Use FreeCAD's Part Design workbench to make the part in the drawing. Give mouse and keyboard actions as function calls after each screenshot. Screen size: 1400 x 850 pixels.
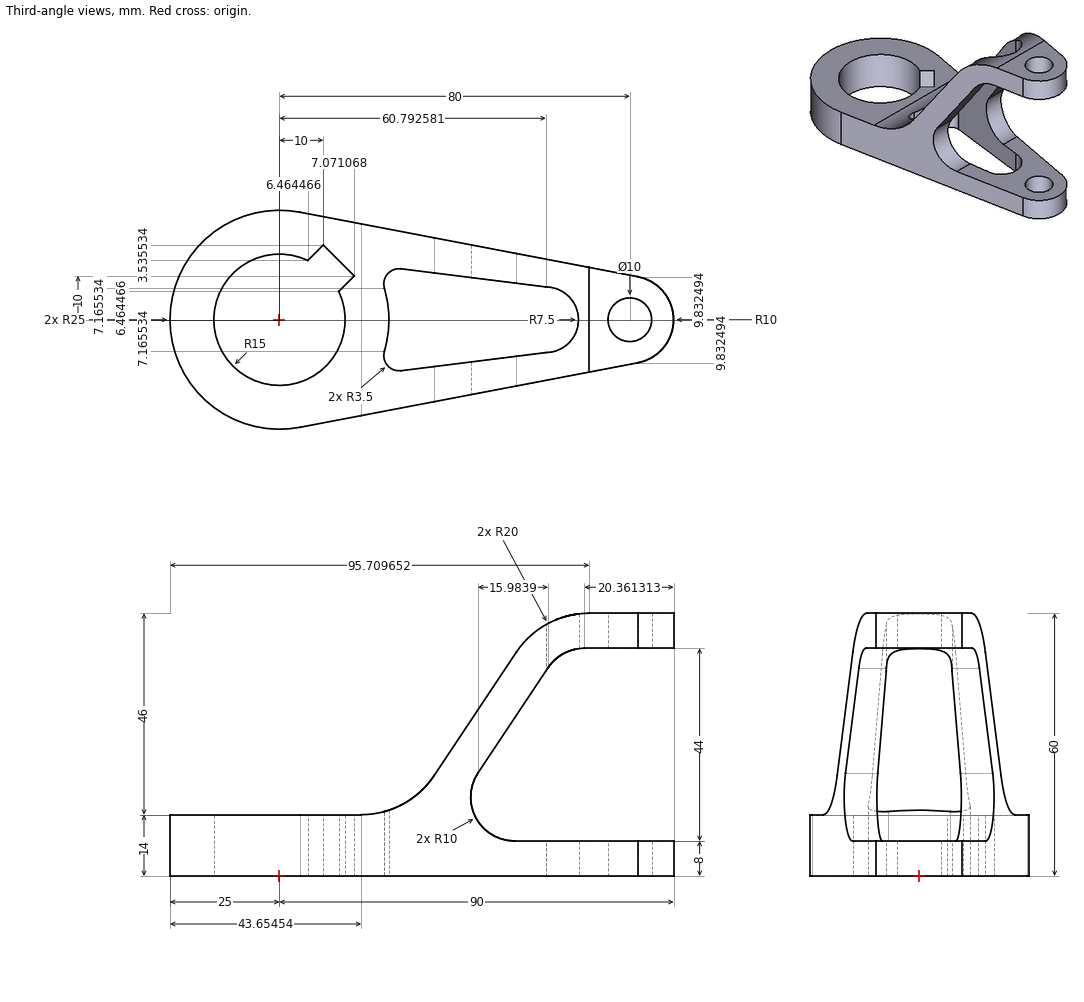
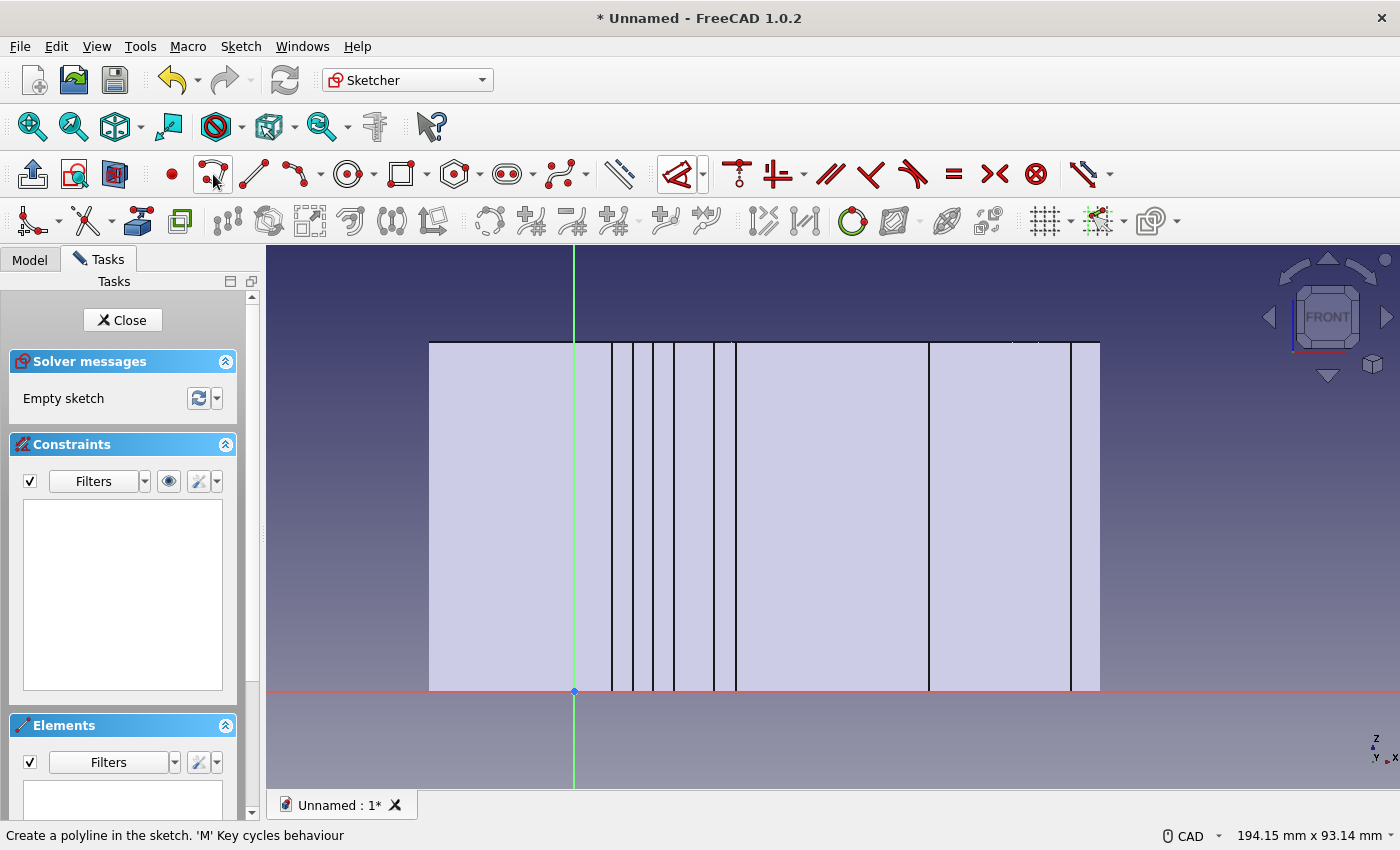
click(683, 610)
click(428, 610)
click(428, 342)
click(987, 342)
right_click(987, 342)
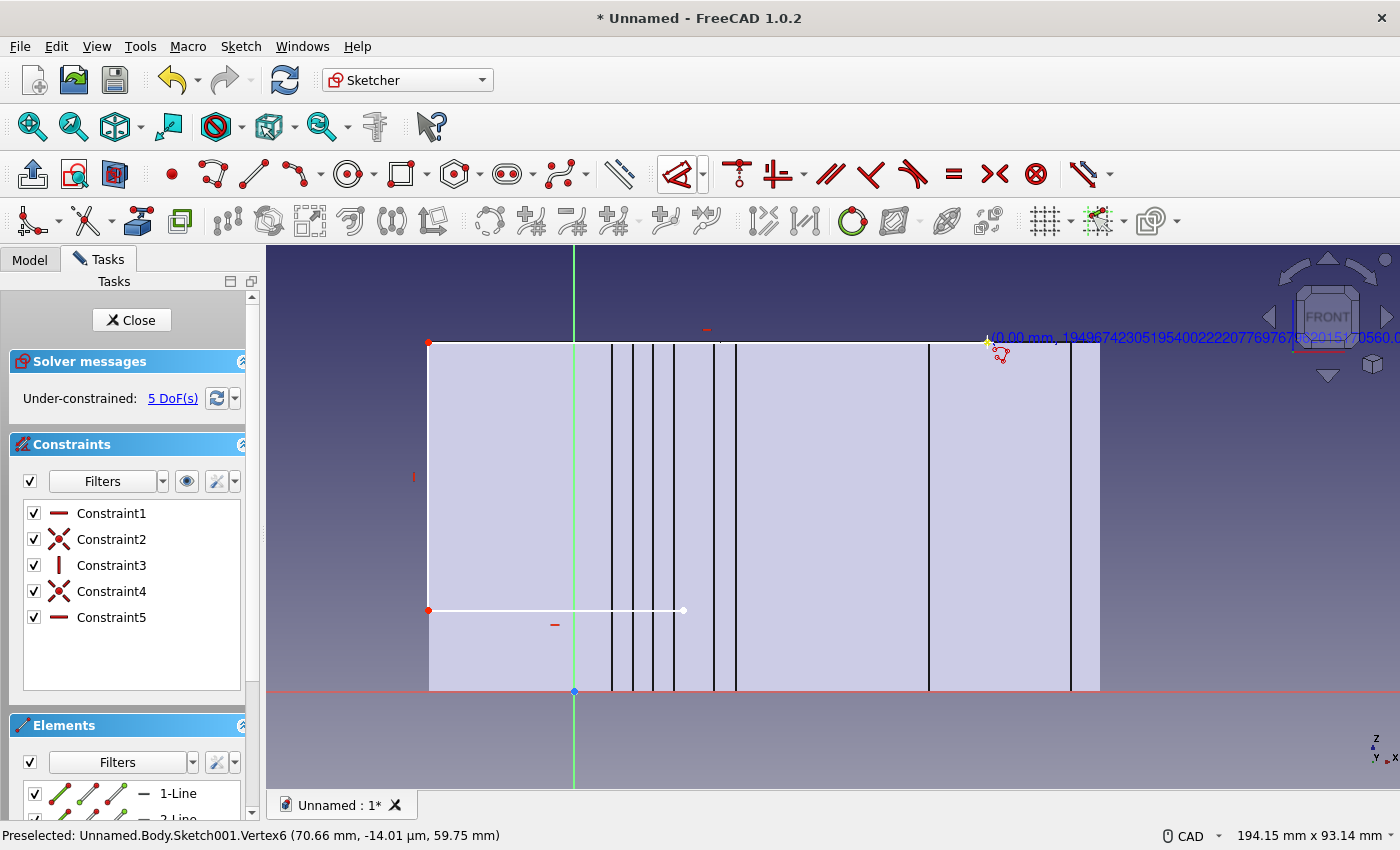
click(254, 174)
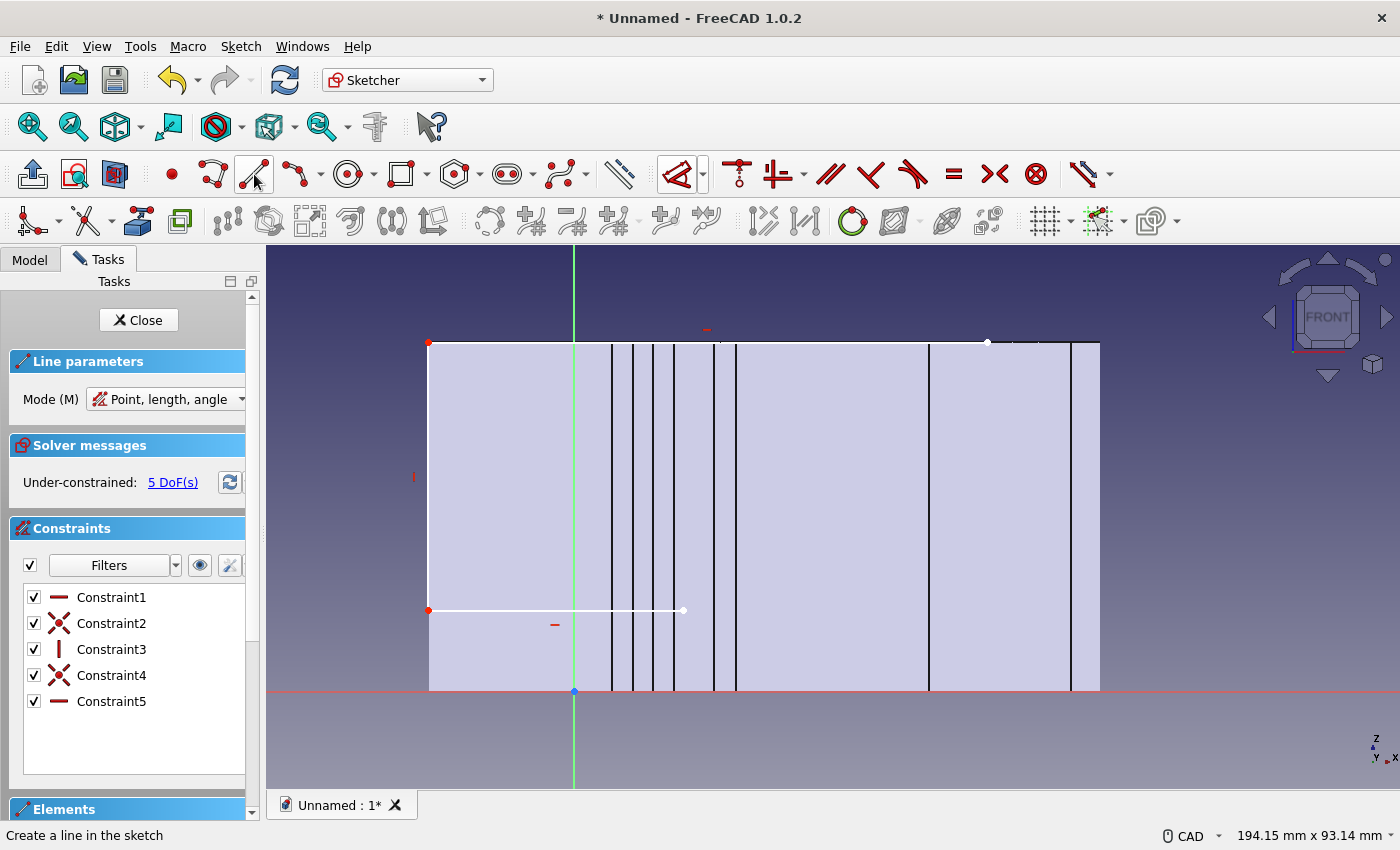
click(890, 394)
click(780, 558)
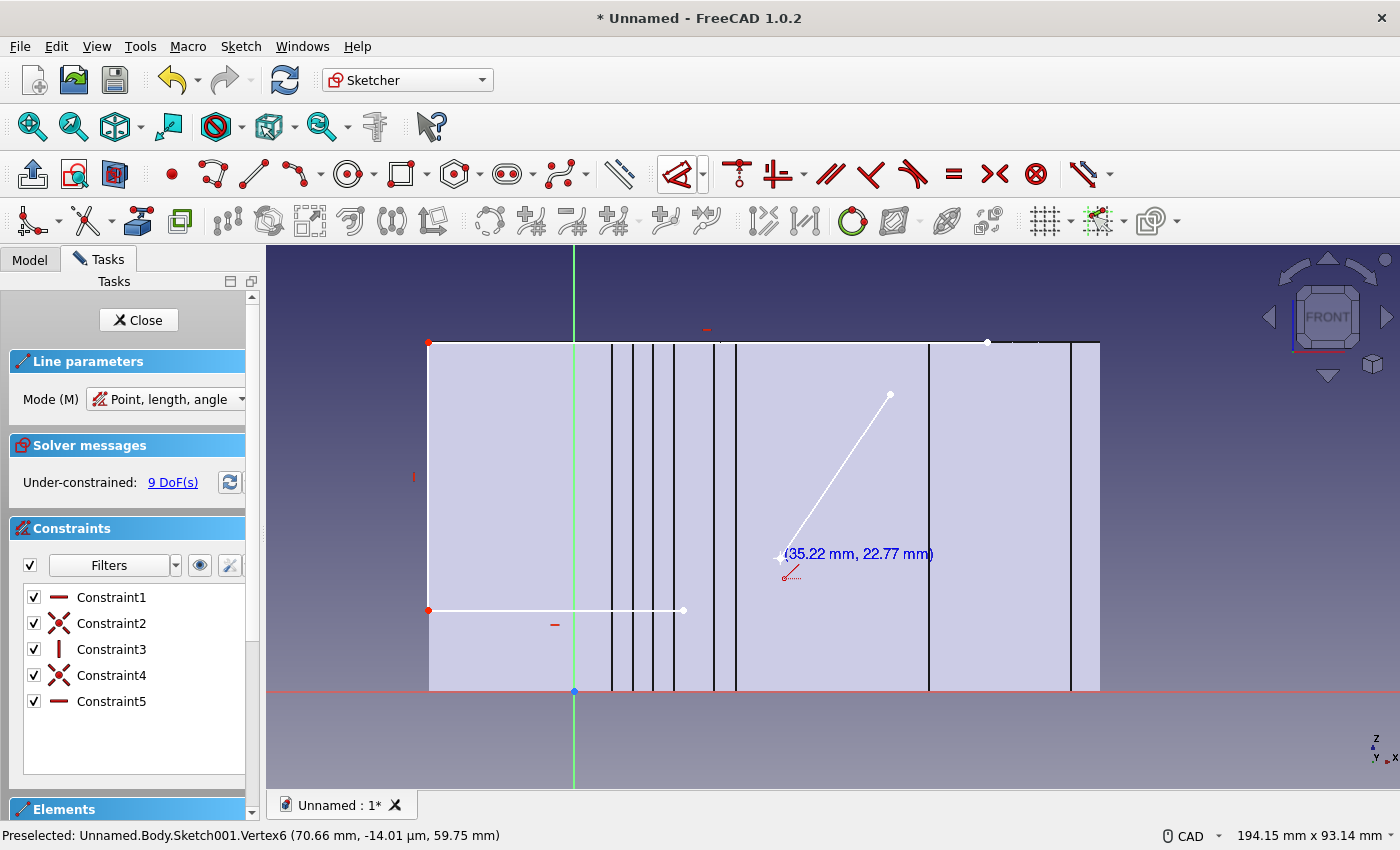
key(g)
key(3)
key(a)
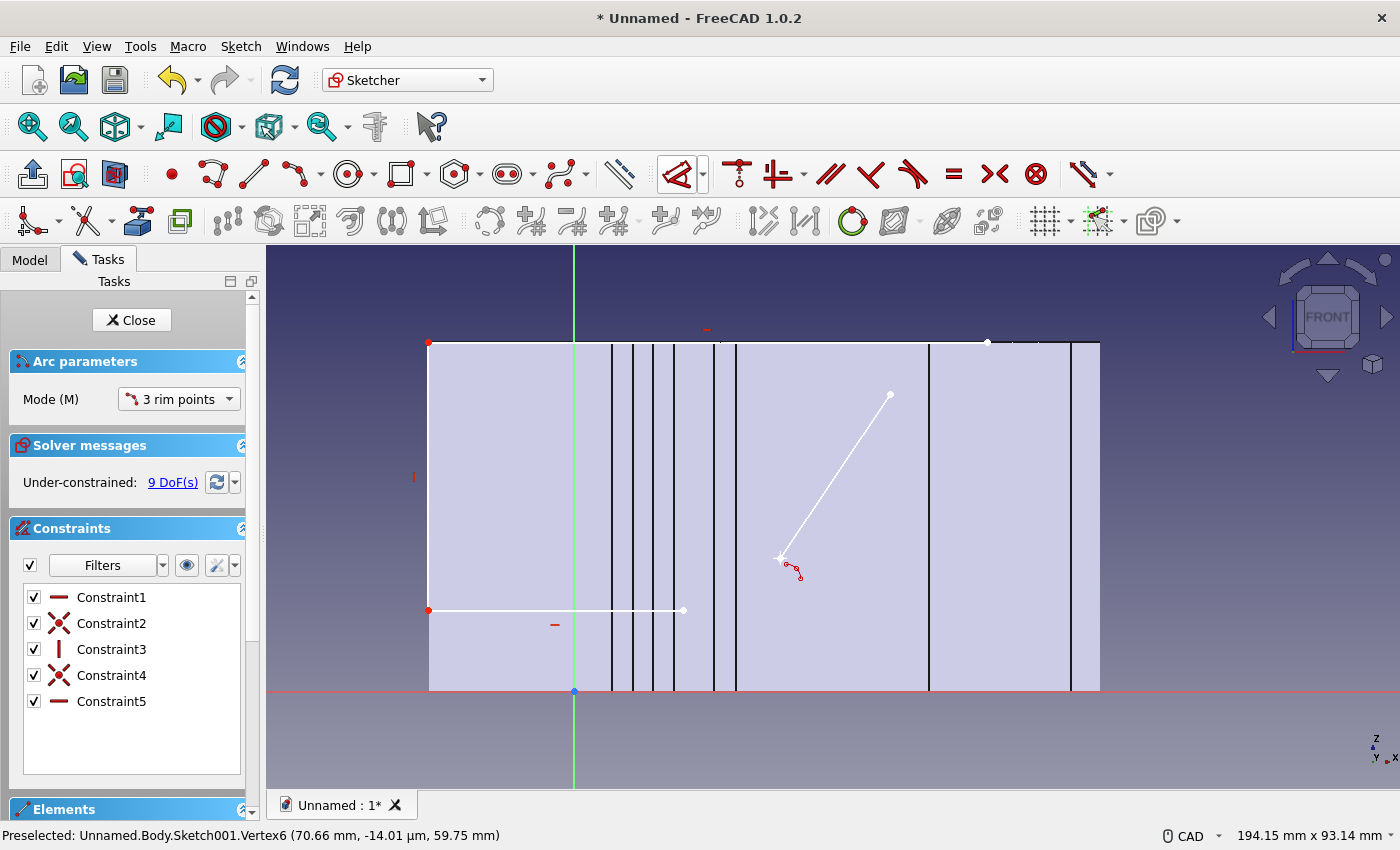
click(987, 343)
click(890, 395)
click(932, 355)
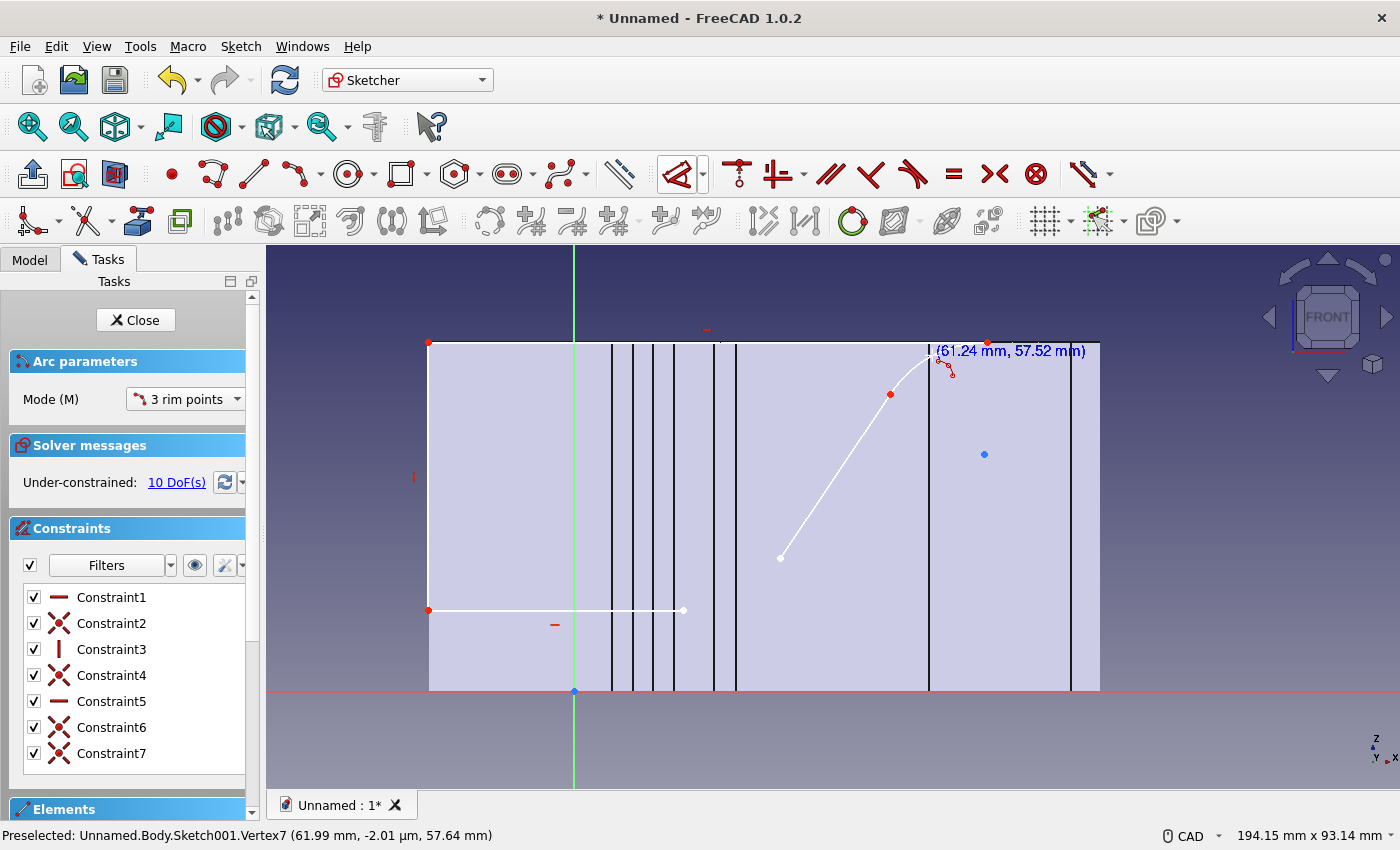
click(780, 559)
click(683, 611)
click(738, 596)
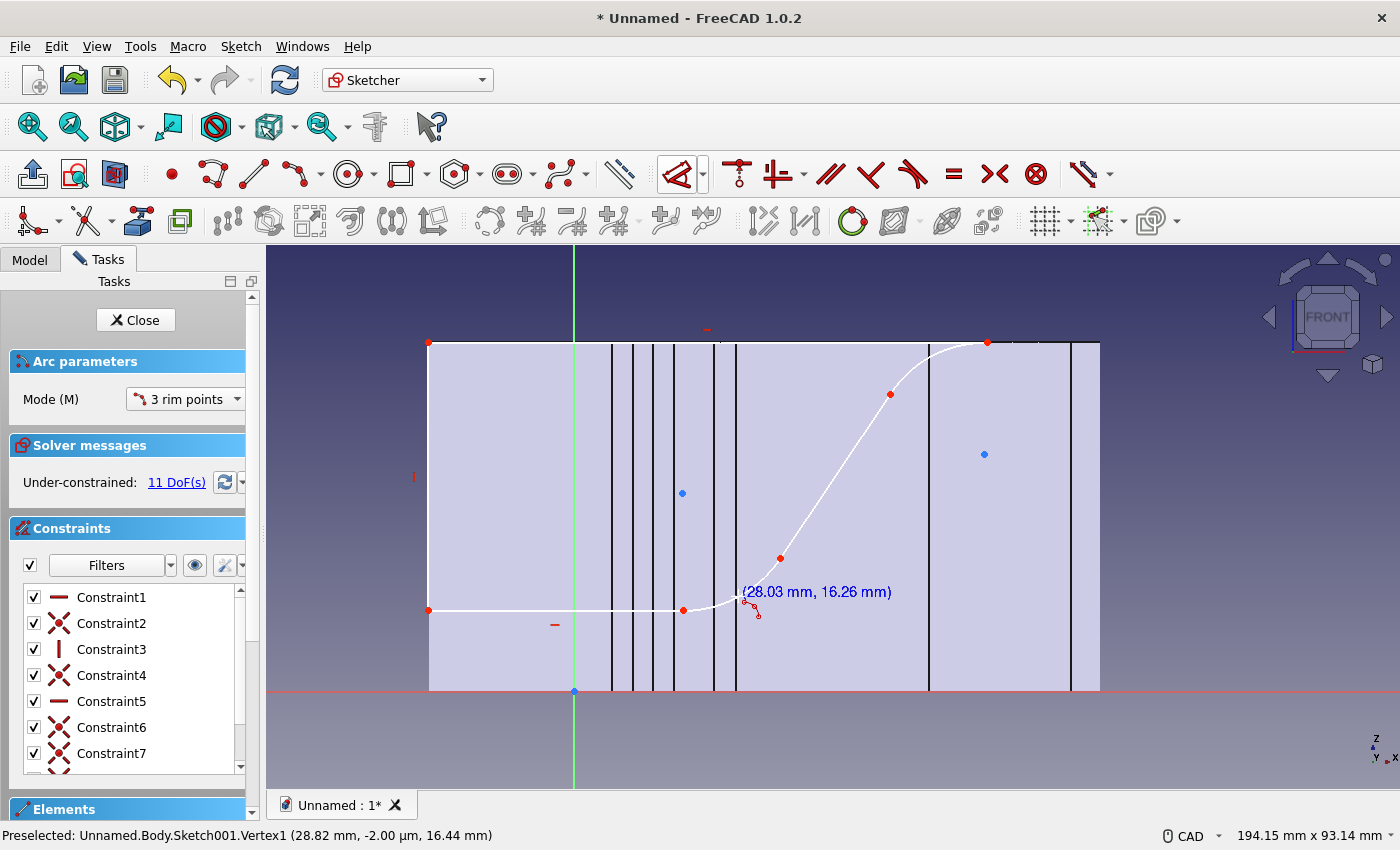
click(254, 174)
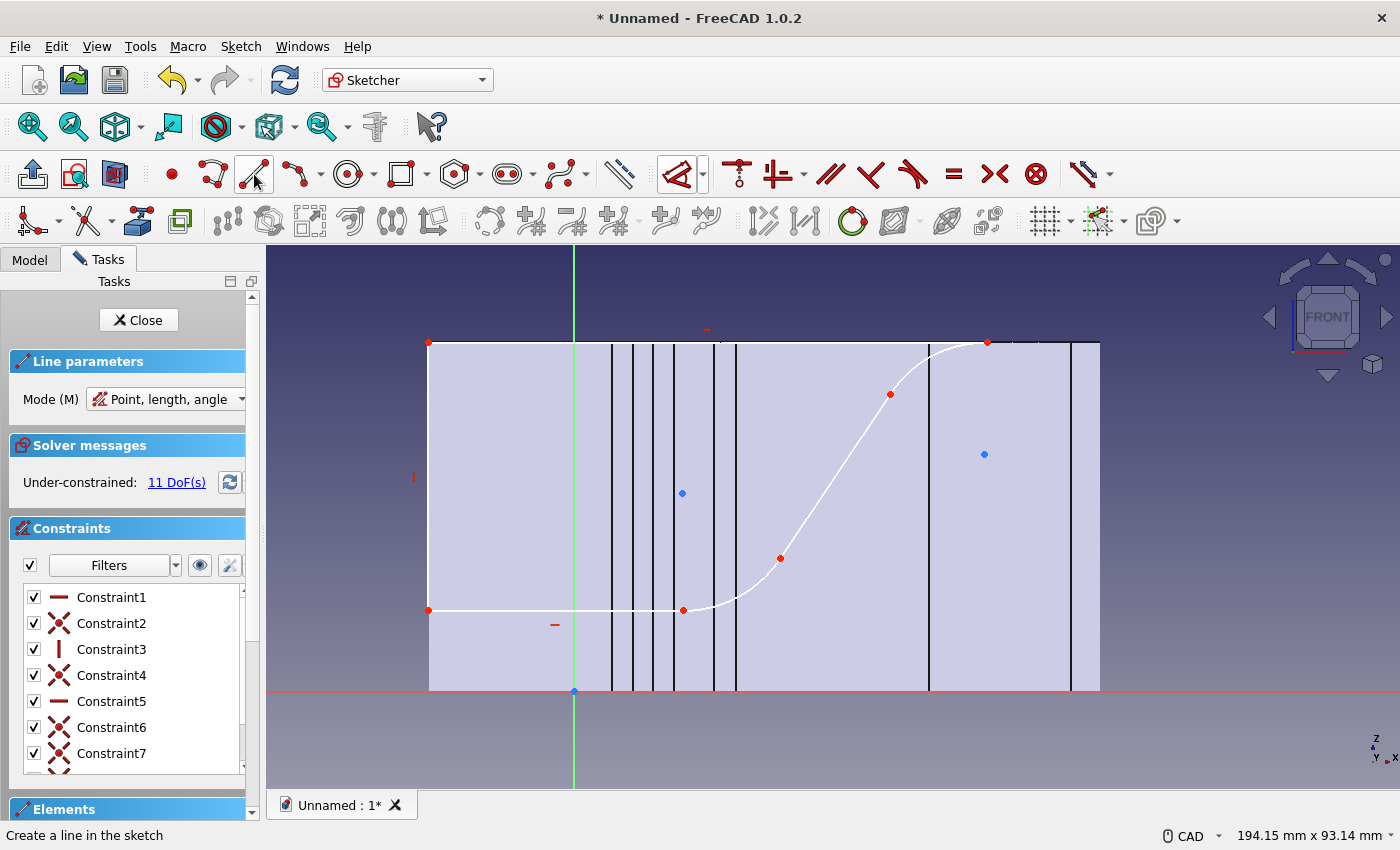
click(839, 554)
click(932, 414)